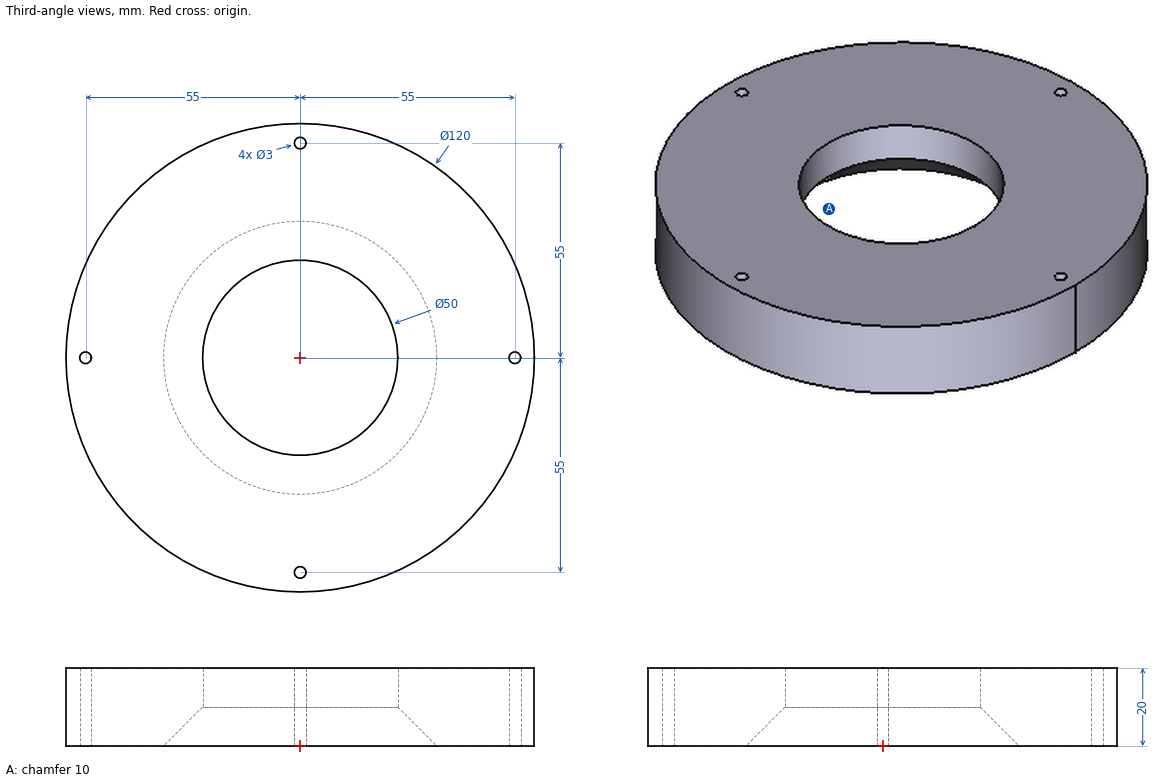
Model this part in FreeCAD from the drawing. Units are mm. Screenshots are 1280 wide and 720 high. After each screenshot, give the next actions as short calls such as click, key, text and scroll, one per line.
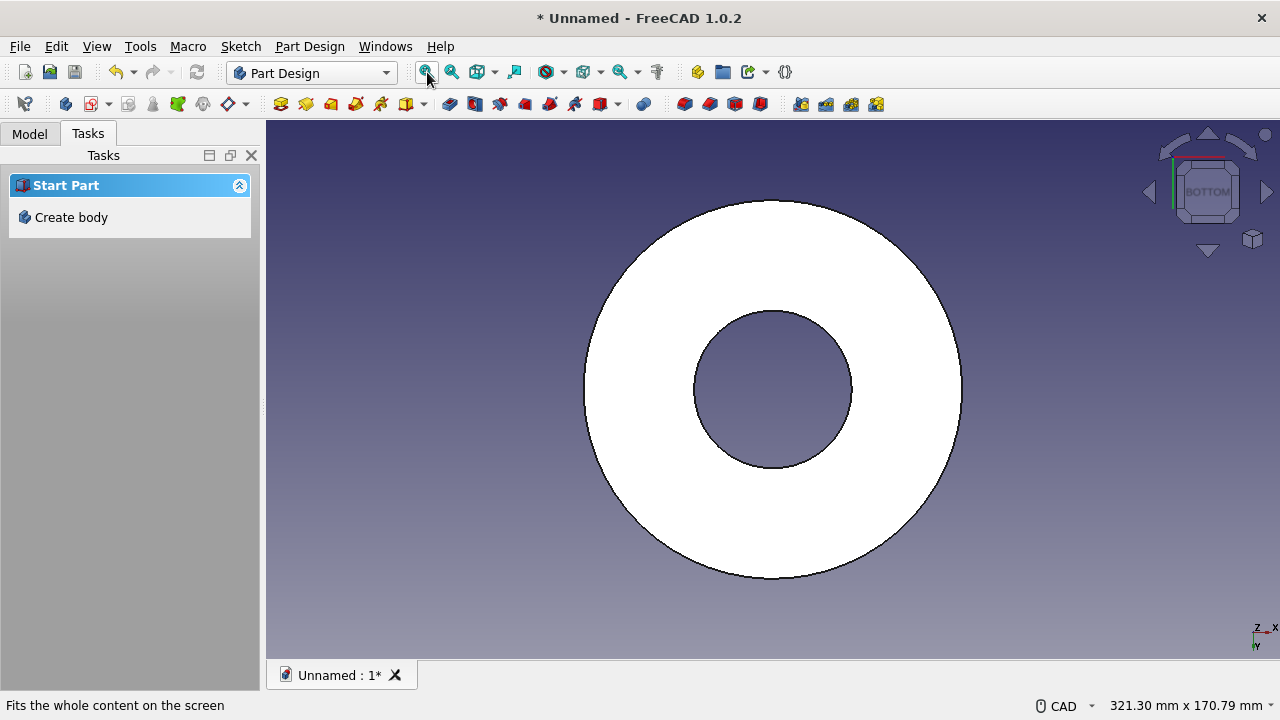
click(694, 388)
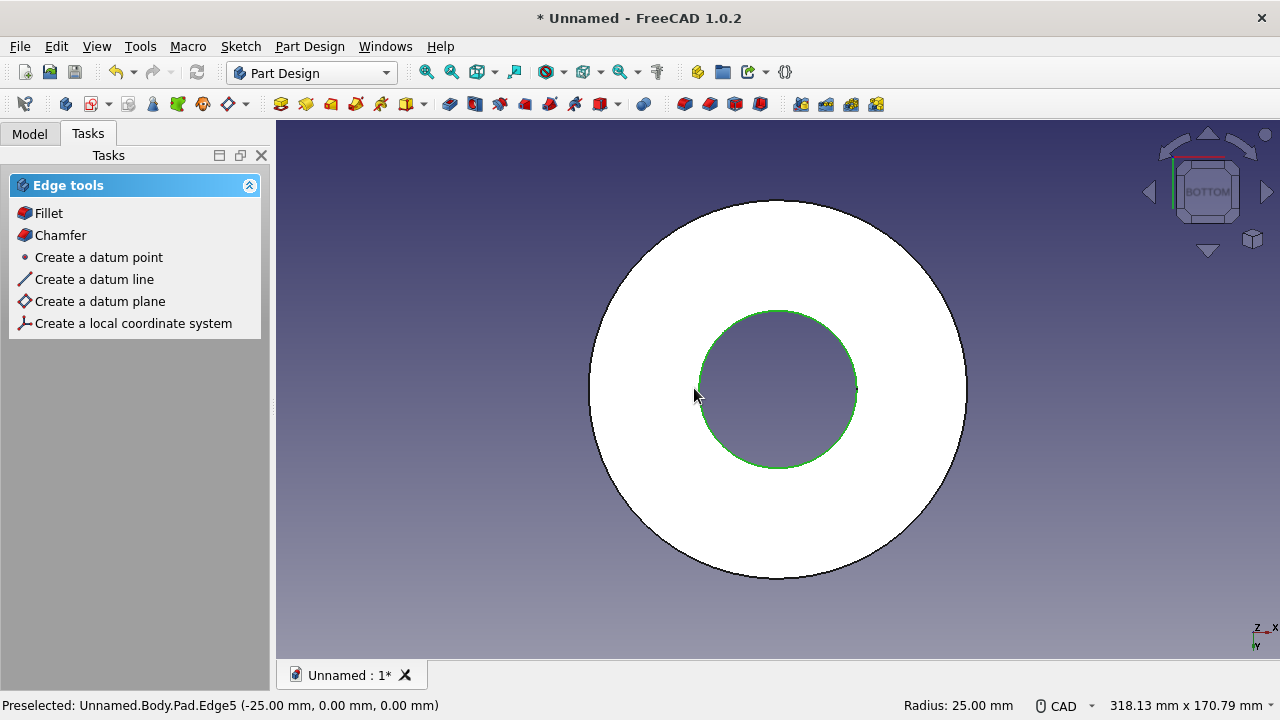
click(710, 104)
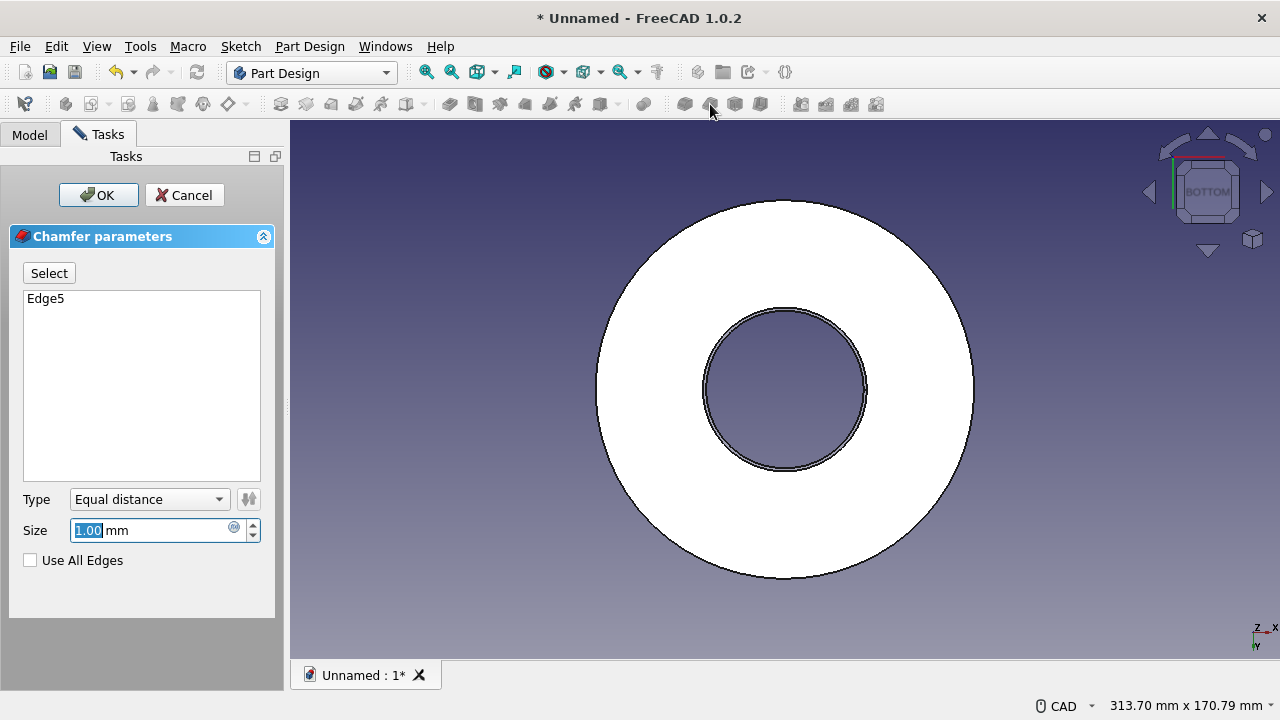
text(10)
key(Tab)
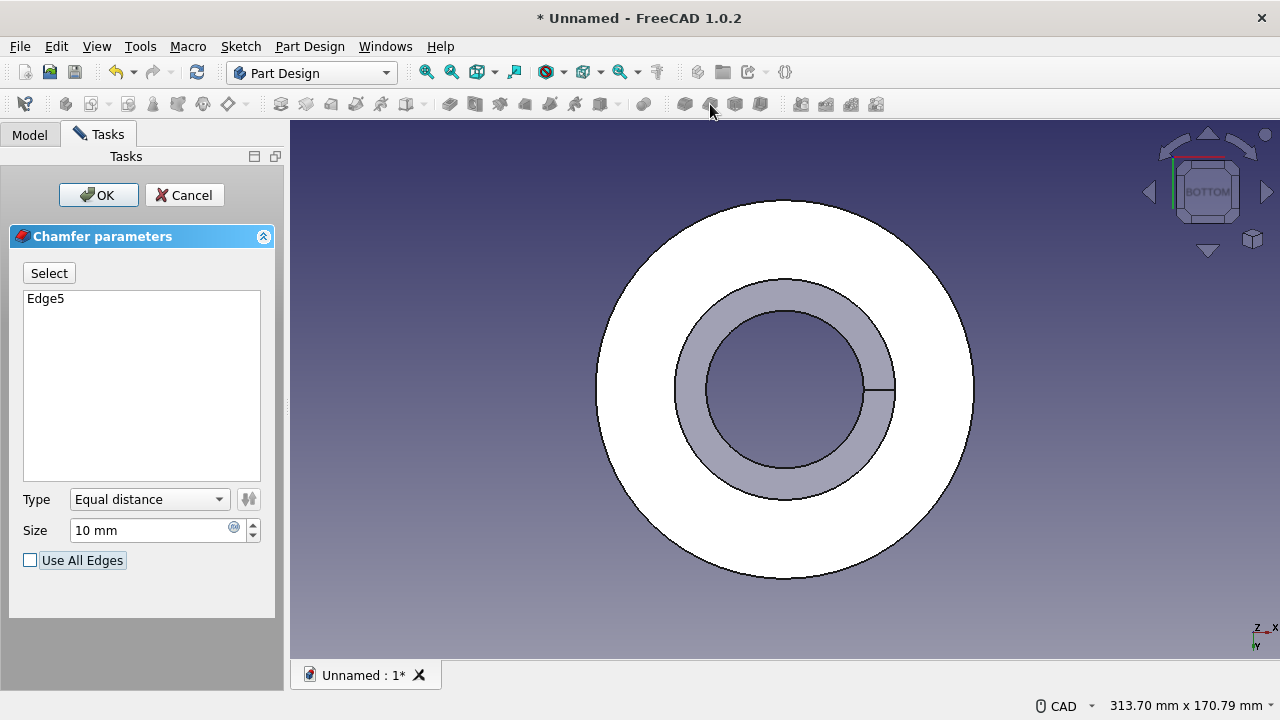
click(99, 195)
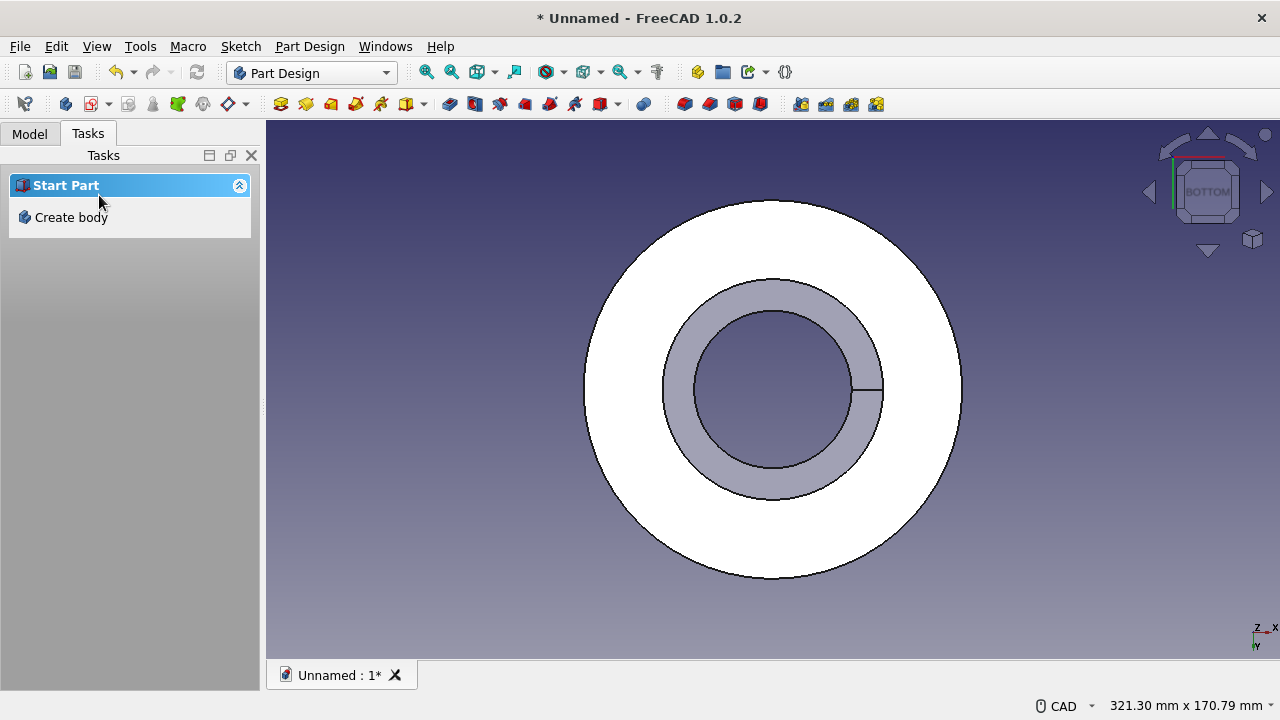
key(0)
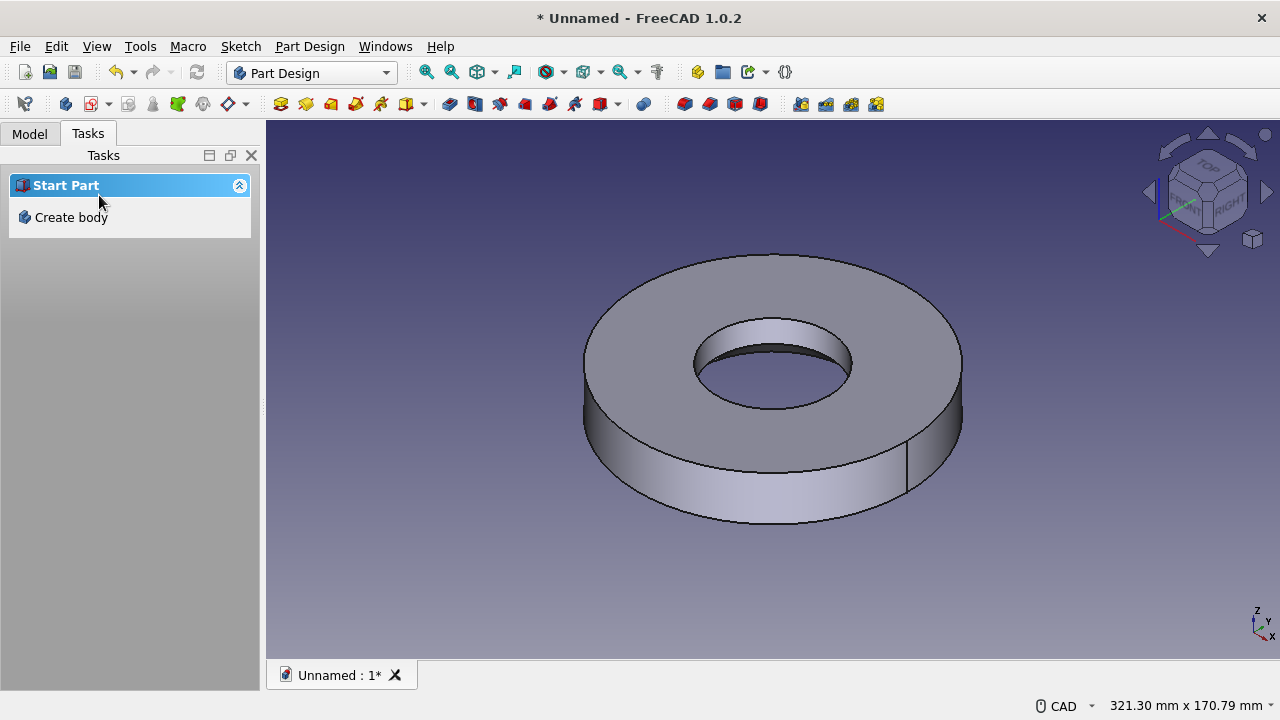
click(811, 296)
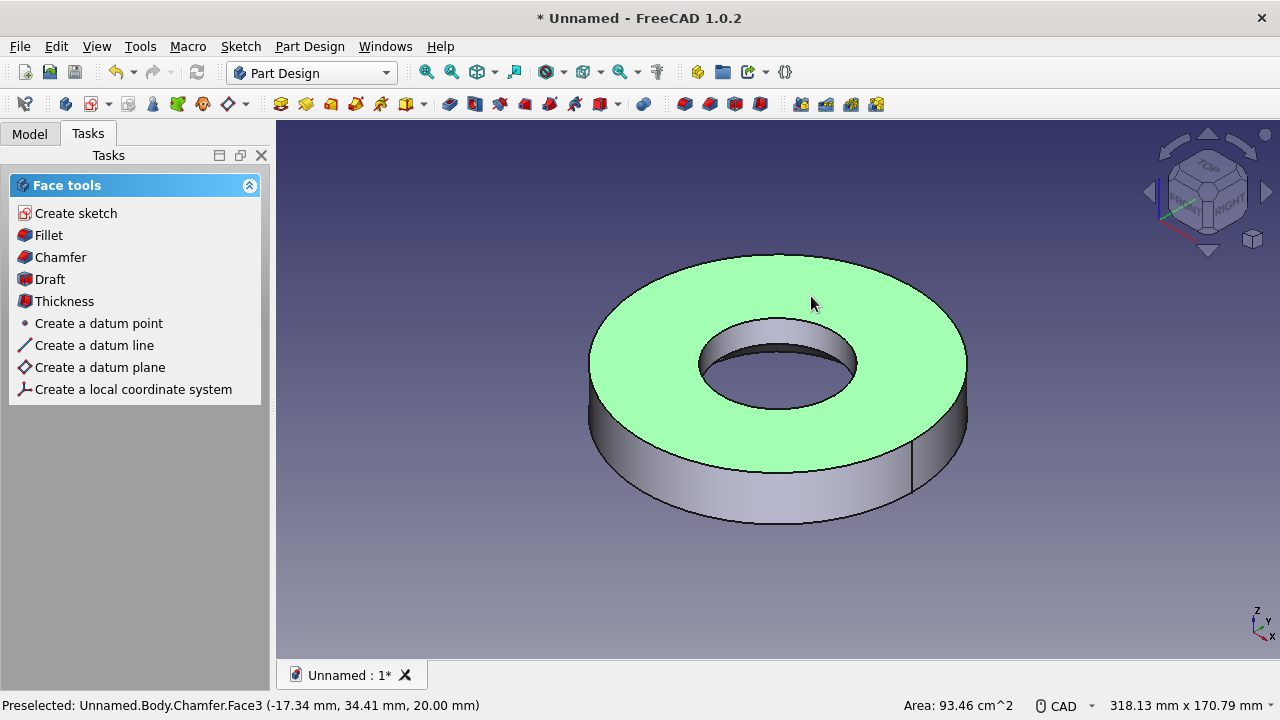
click(90, 104)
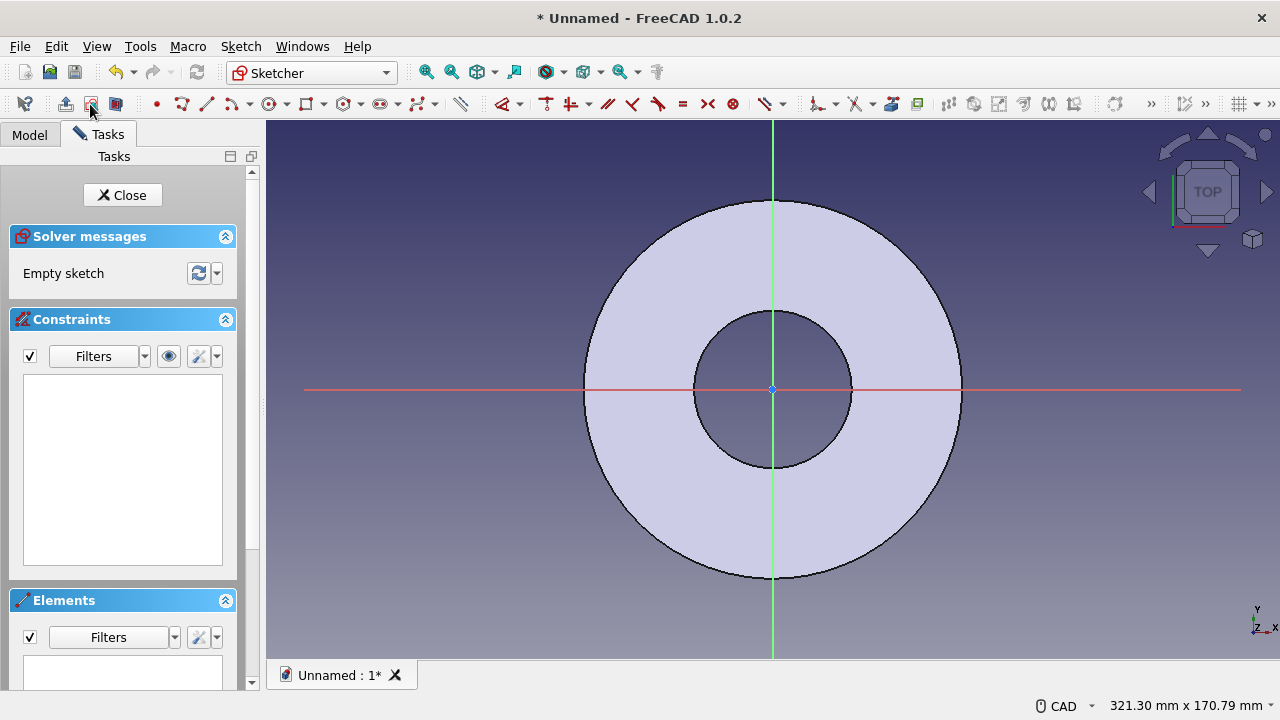
key(g)
key(c)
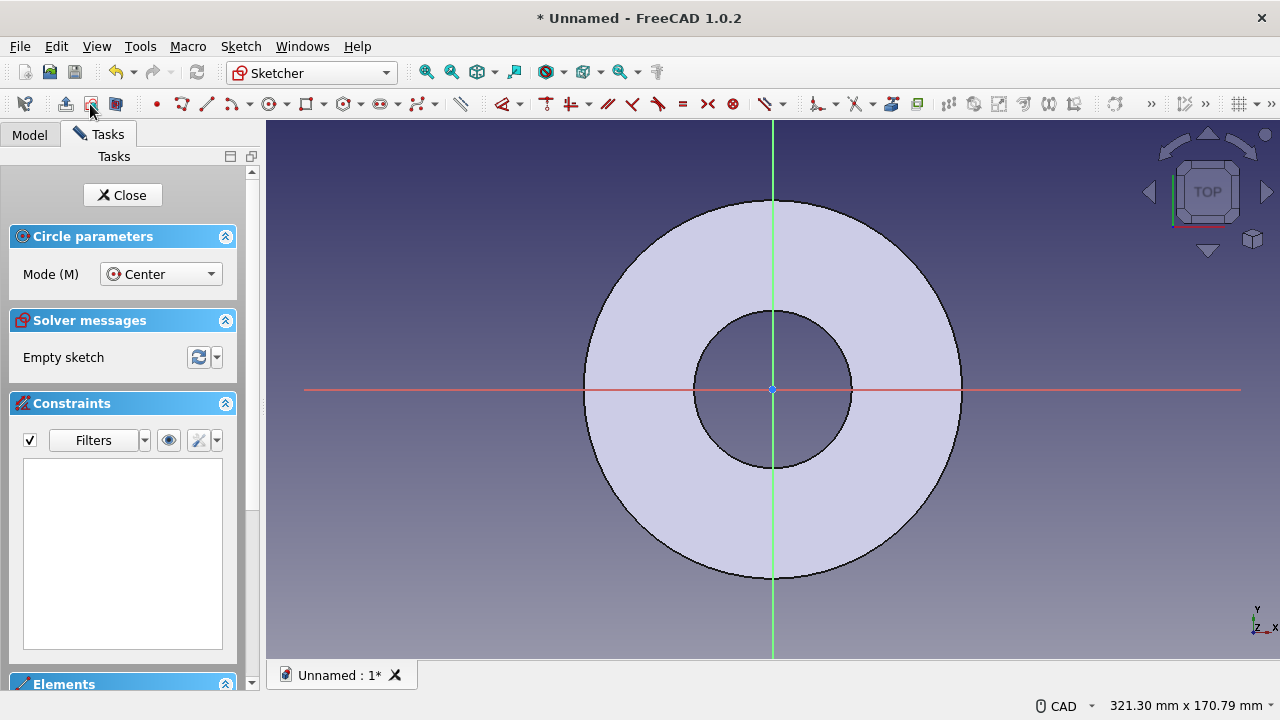
scroll(773, 216, up, 8)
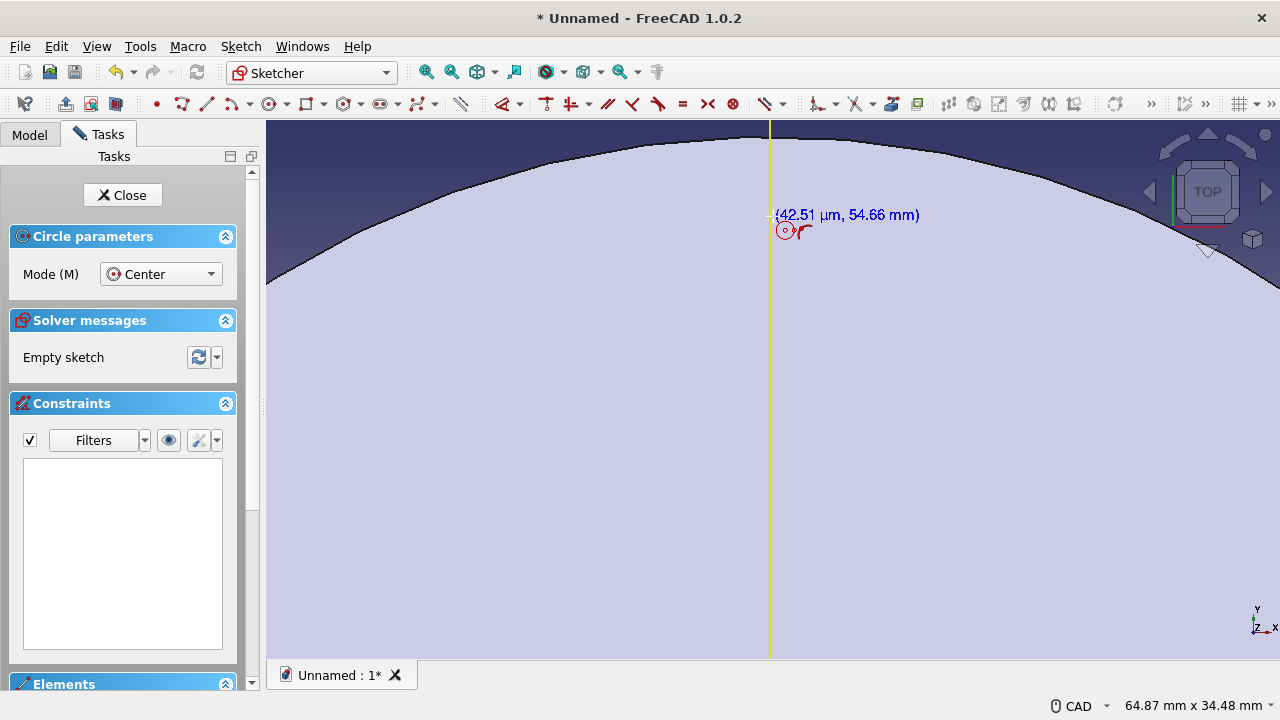
scroll(688, 216, down, 8)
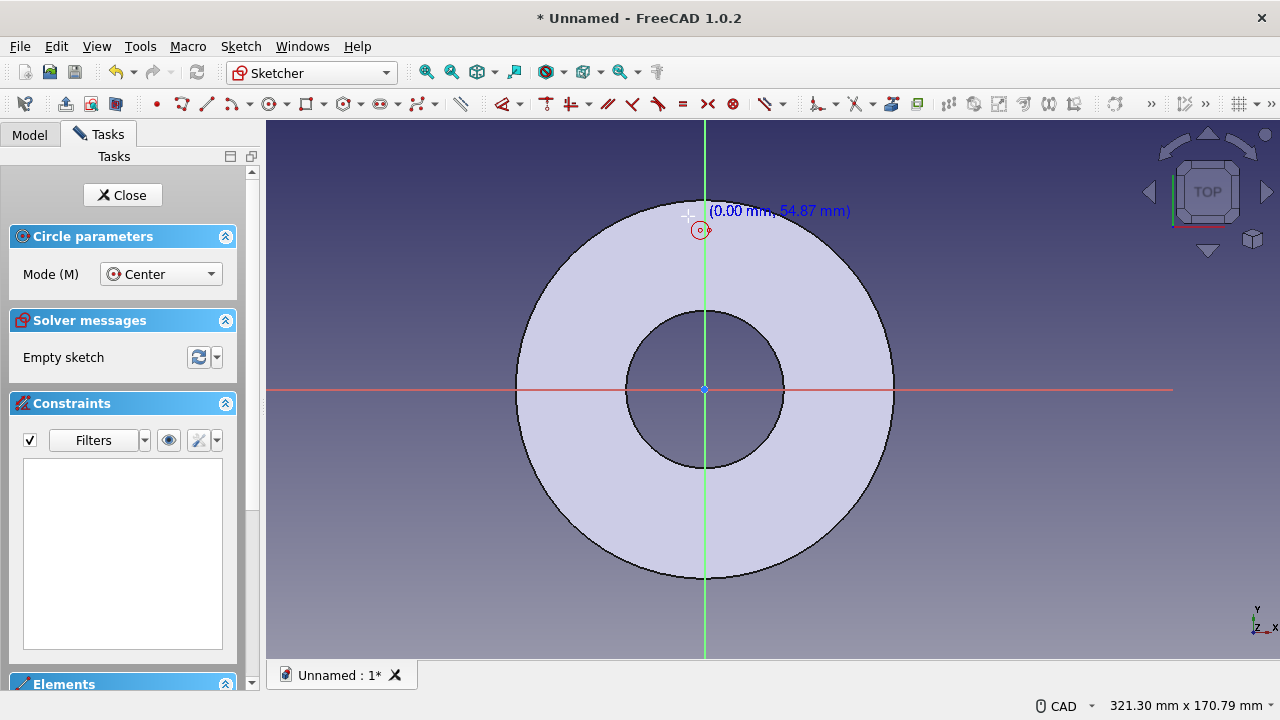
click(705, 216)